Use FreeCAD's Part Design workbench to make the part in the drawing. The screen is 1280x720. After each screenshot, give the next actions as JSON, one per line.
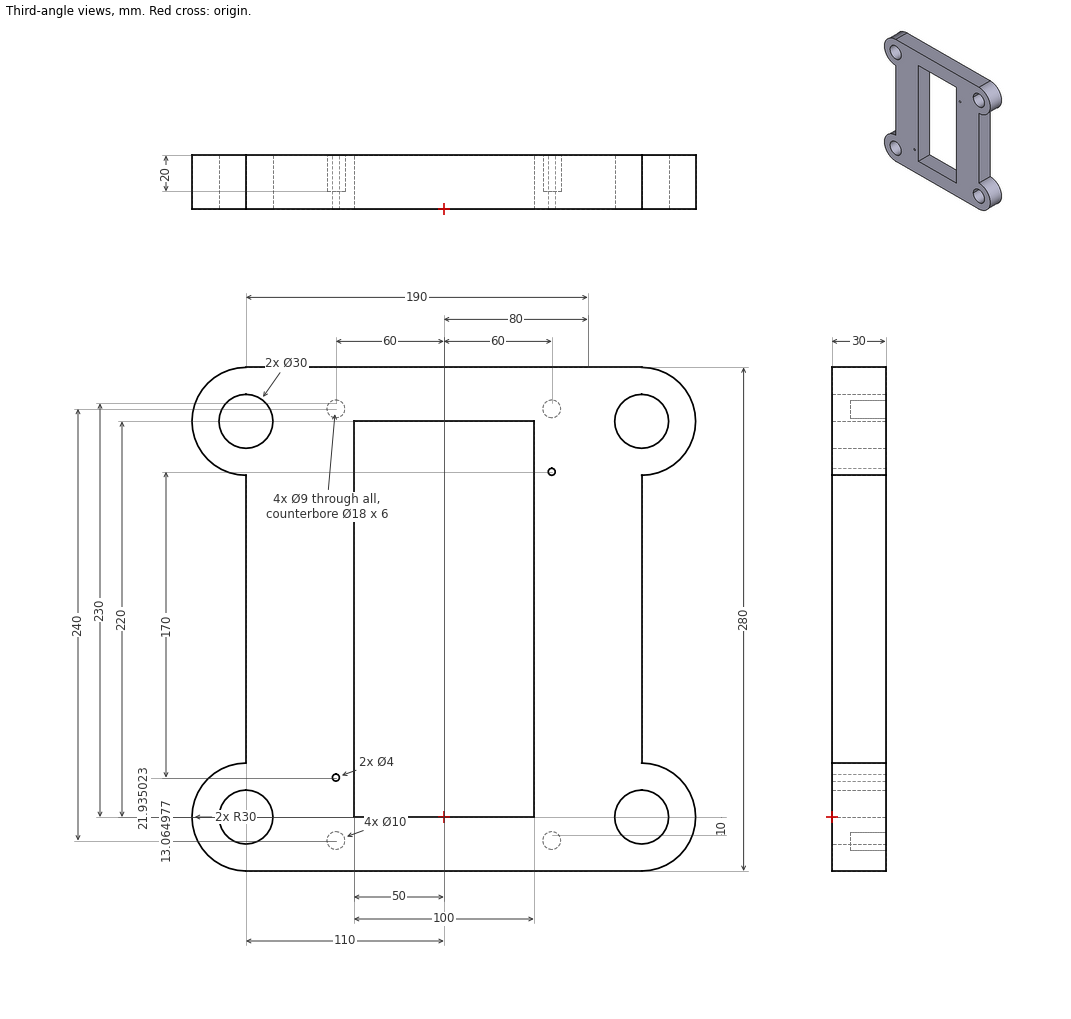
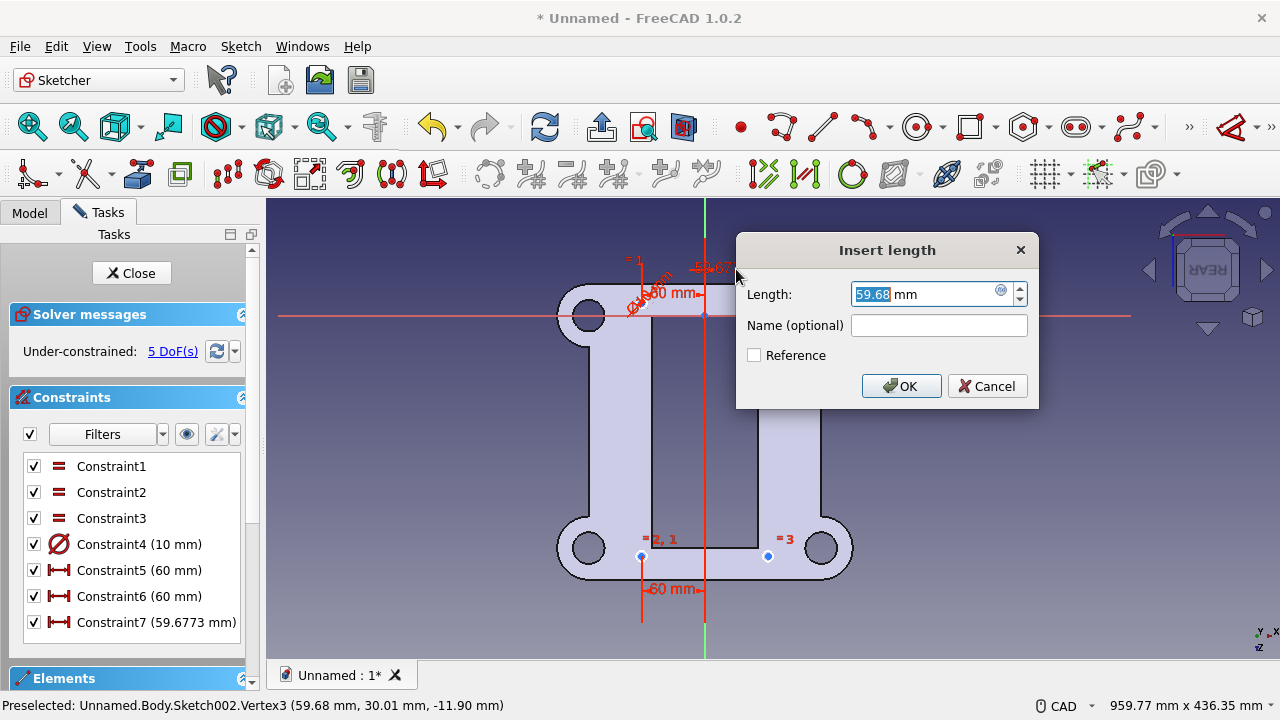
{"action": "type", "text": "60"}
{"action": "key", "text": "Return"}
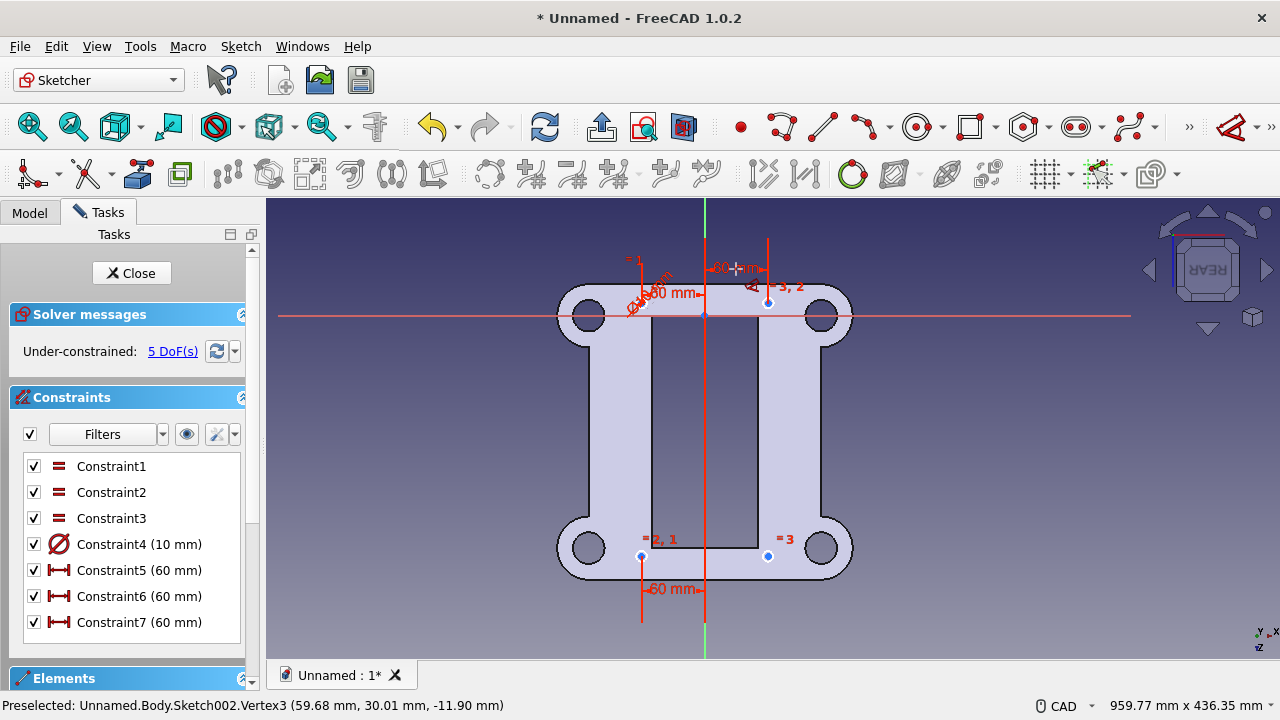
{"action": "left_click", "coordinate": [768, 556]}
{"action": "left_click", "coordinate": [751, 590]}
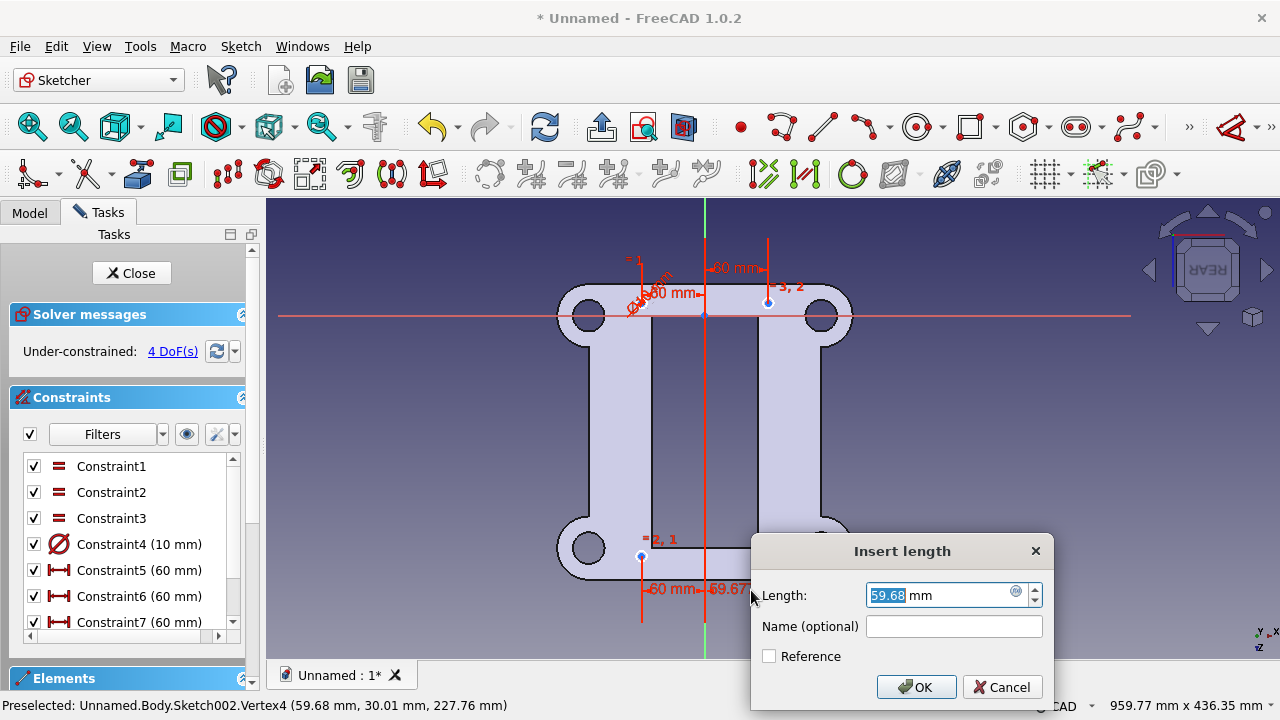
{"action": "type", "text": "60"}
{"action": "key", "text": "Return"}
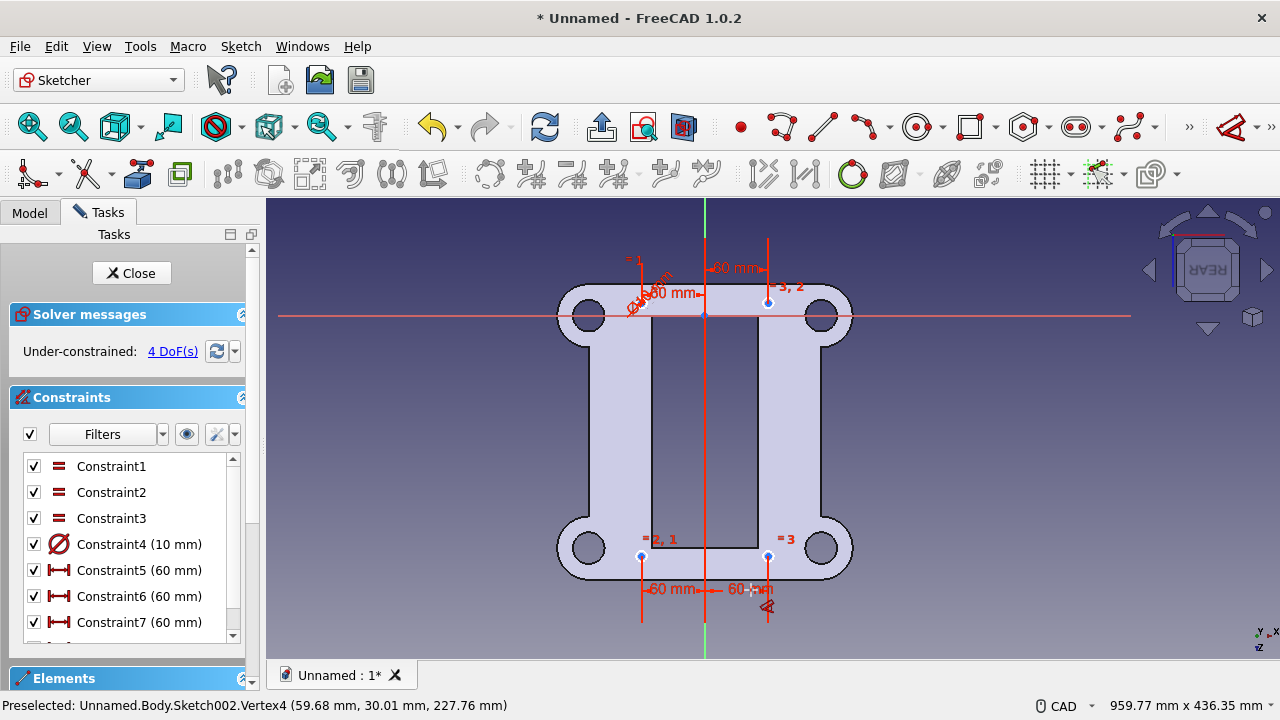
{"action": "left_click", "coordinate": [642, 303]}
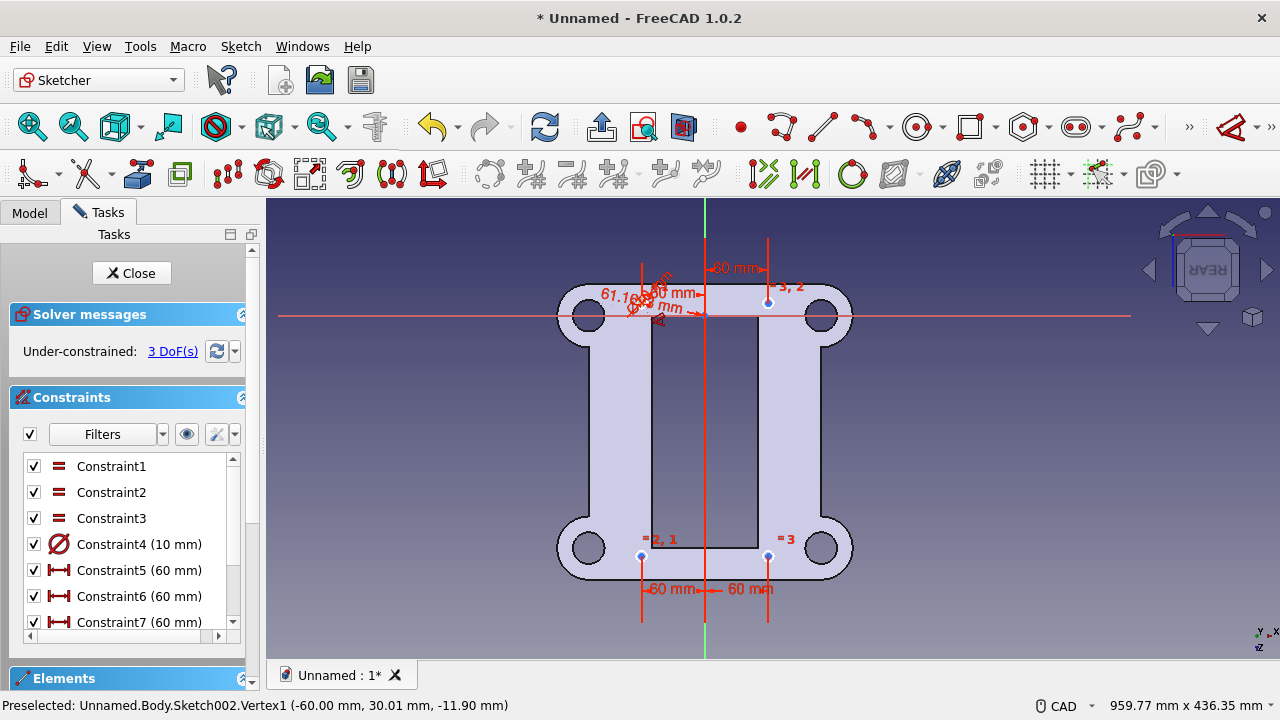
{"action": "left_click", "coordinate": [642, 556]}
{"action": "left_click", "coordinate": [608, 430]}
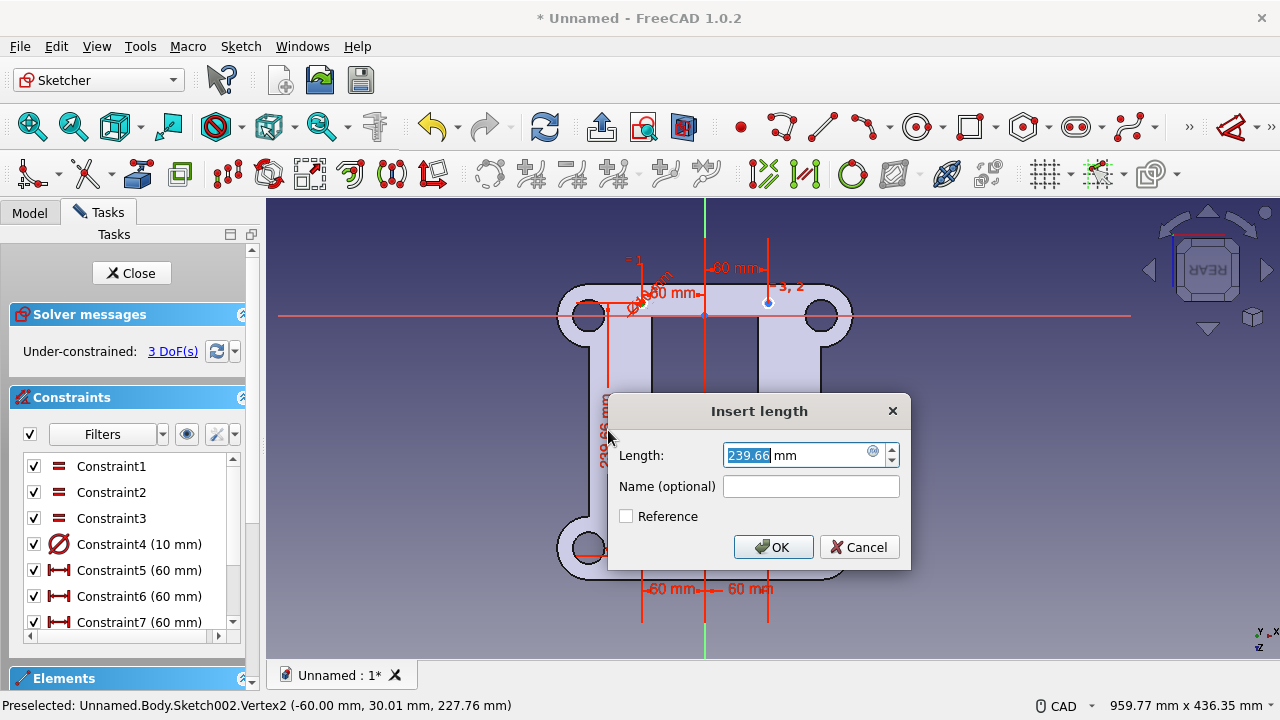
{"action": "type", "text": "240"}
{"action": "key", "text": "Return"}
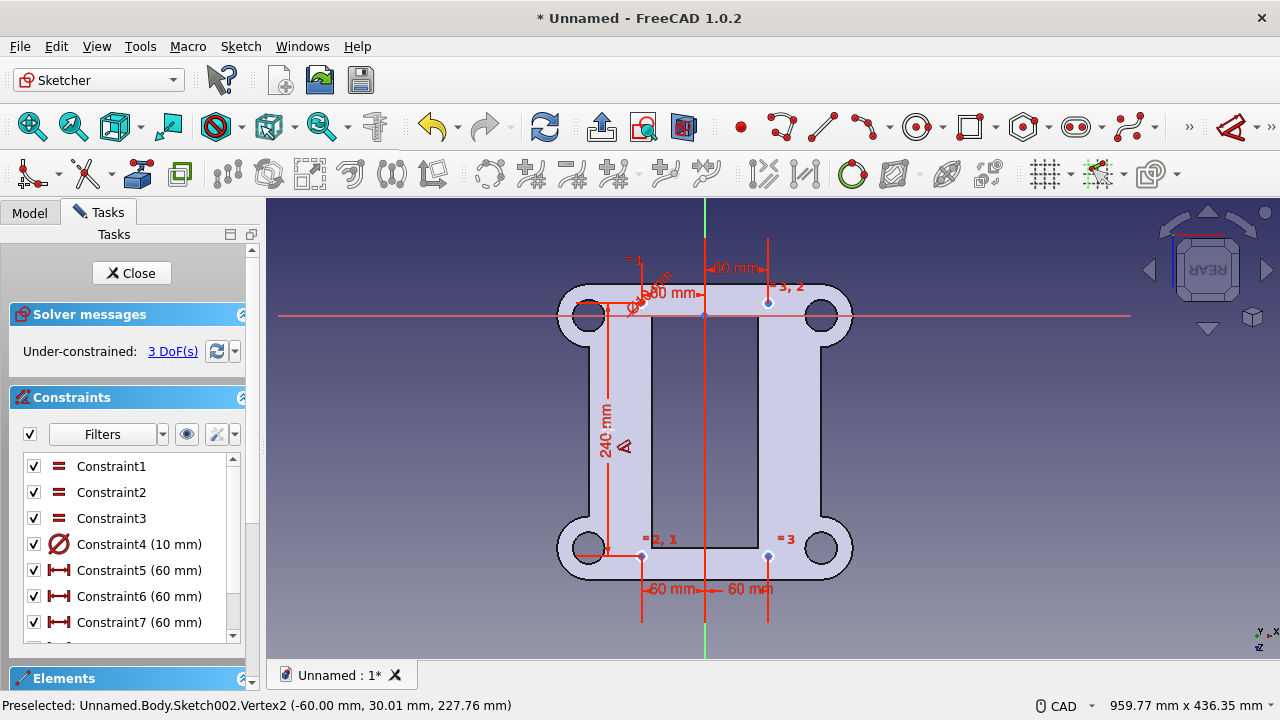
{"action": "left_click", "coordinate": [642, 556]}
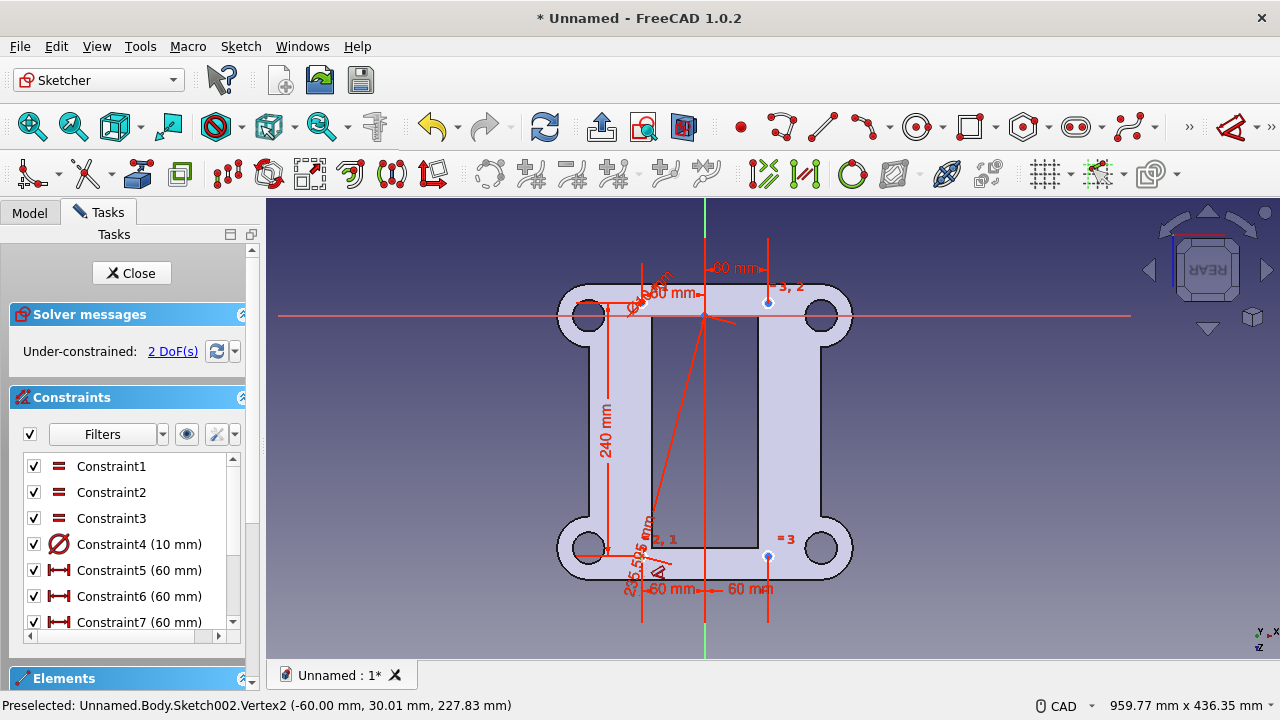
{"action": "left_click", "coordinate": [768, 303]}
{"action": "left_click", "coordinate": [802, 430]}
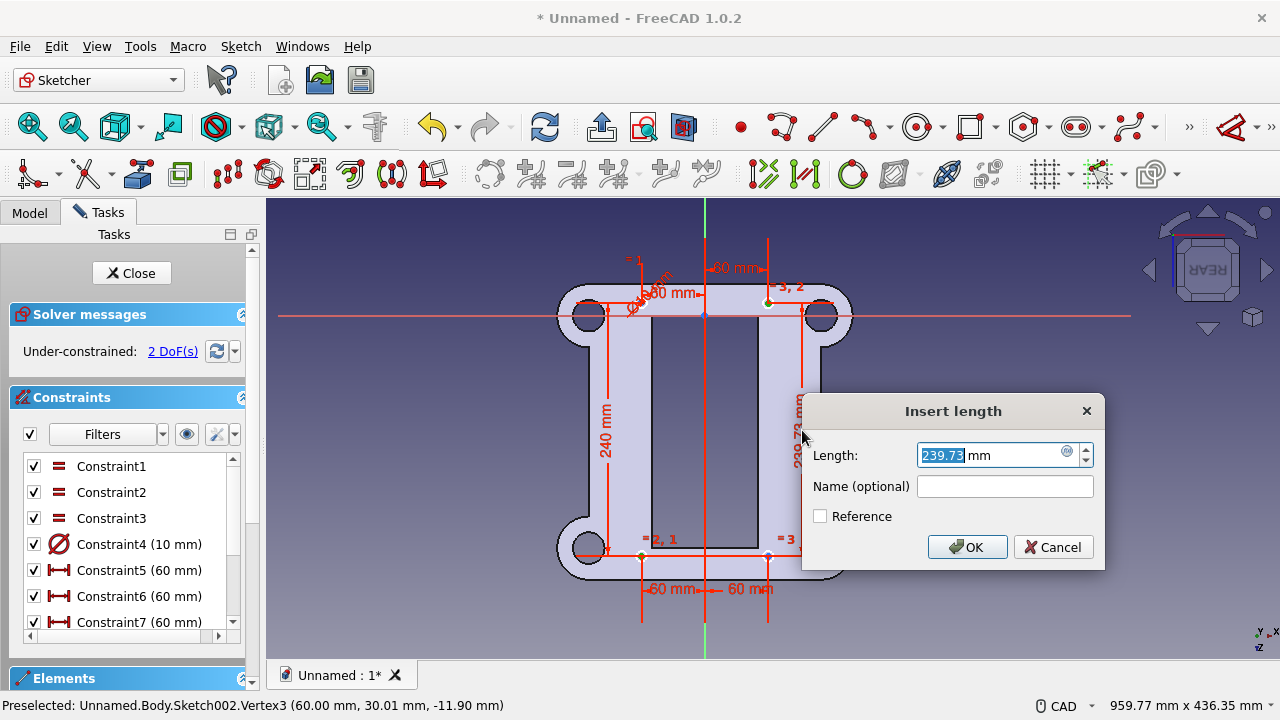
{"action": "type", "text": "240"}
{"action": "key", "text": "Return"}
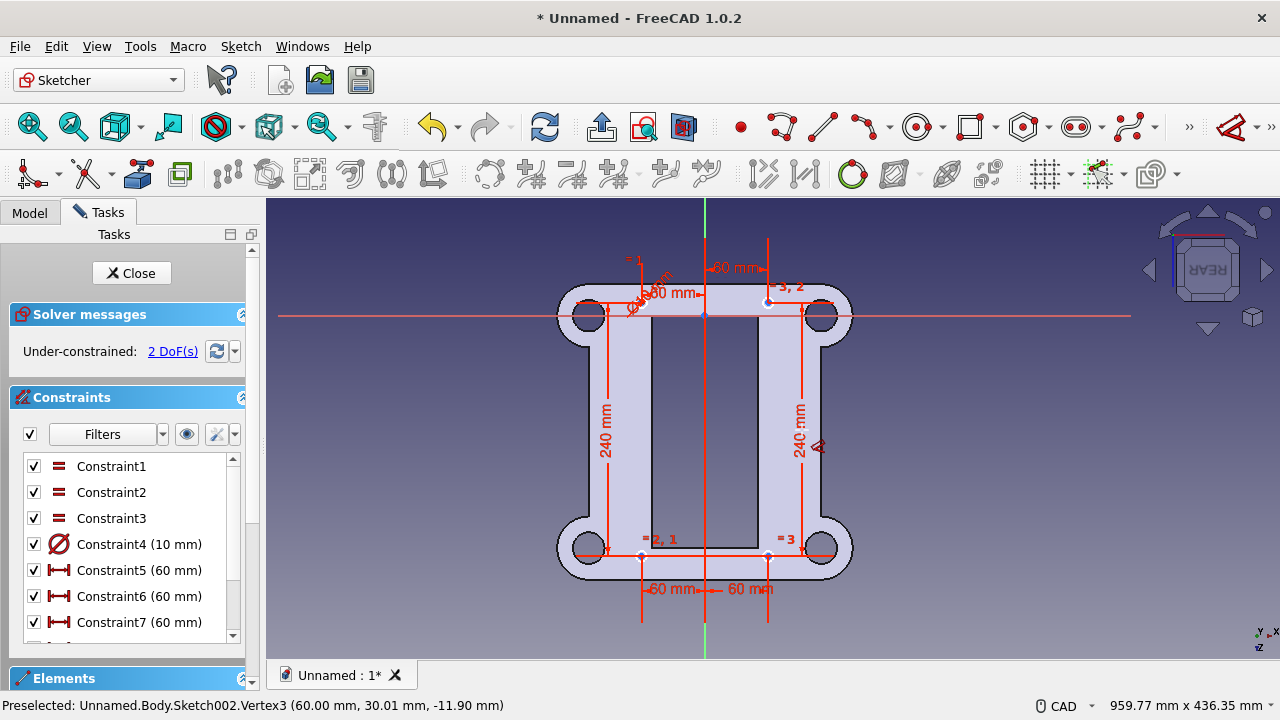
{"action": "left_click", "coordinate": [768, 303]}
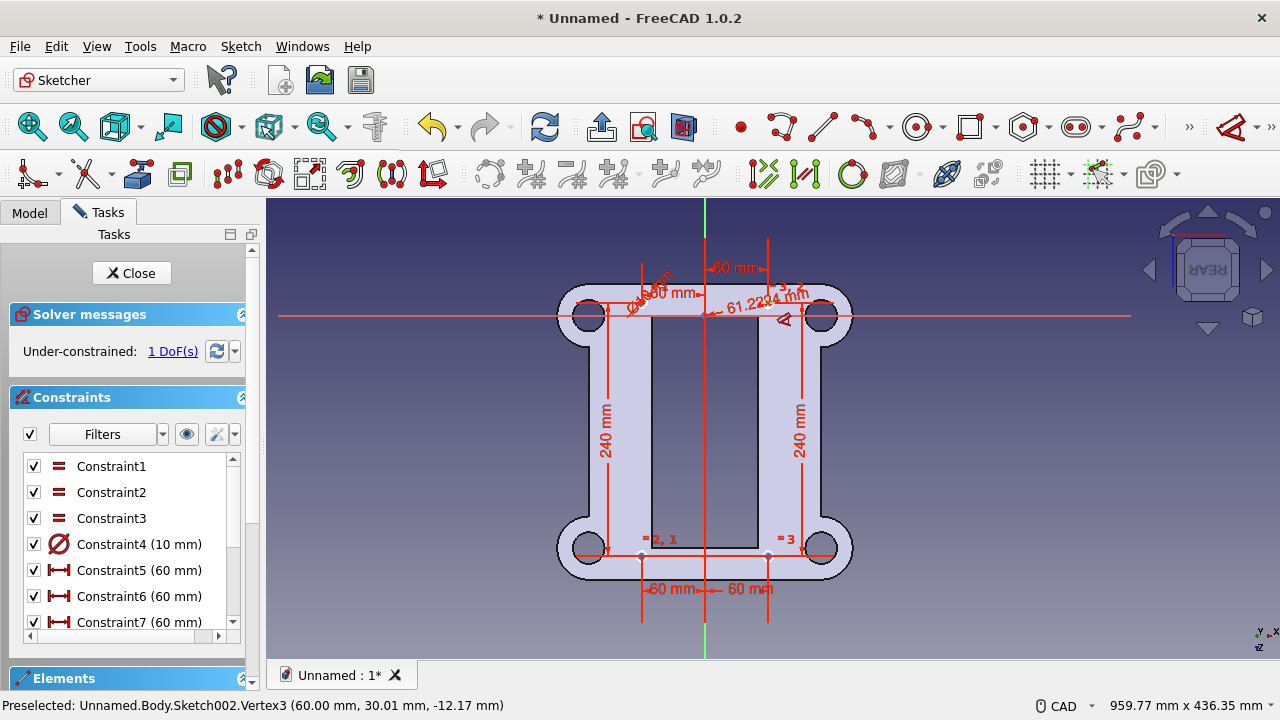
{"action": "left_click", "coordinate": [768, 556]}
{"action": "left_click", "coordinate": [802, 371]}